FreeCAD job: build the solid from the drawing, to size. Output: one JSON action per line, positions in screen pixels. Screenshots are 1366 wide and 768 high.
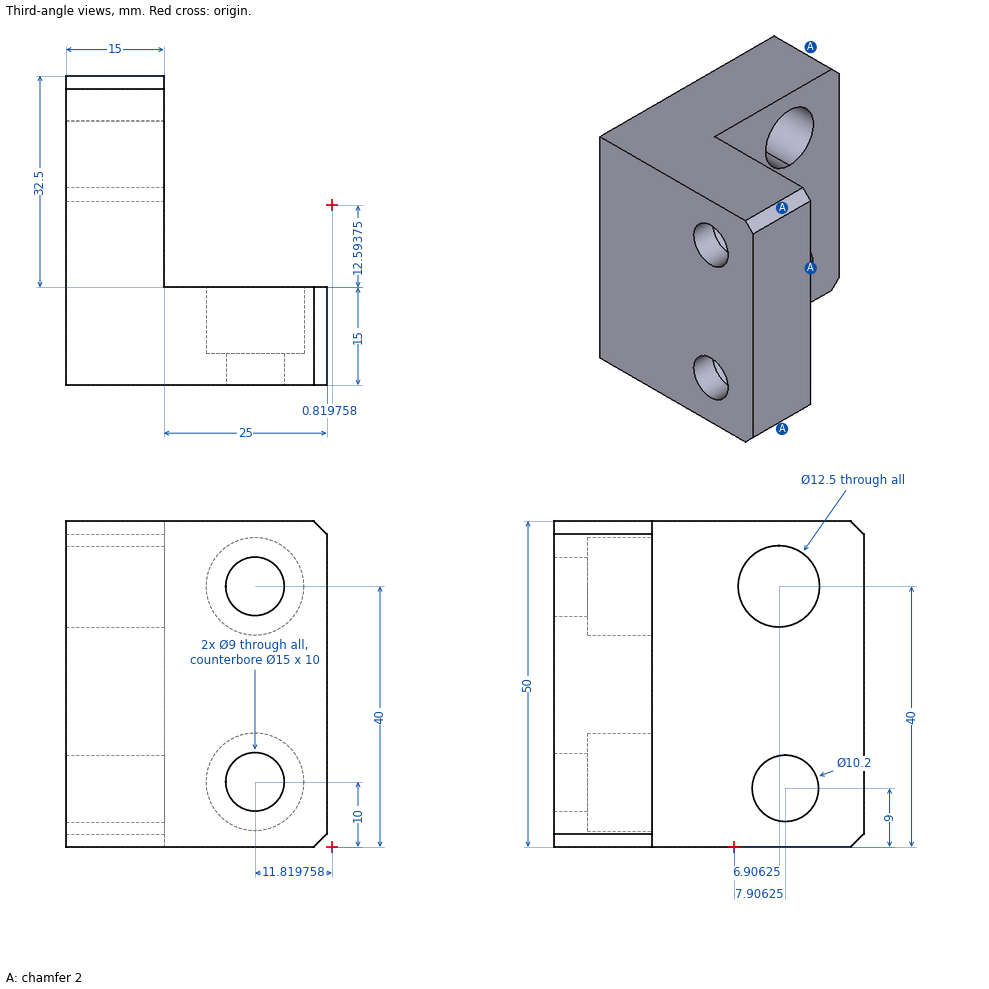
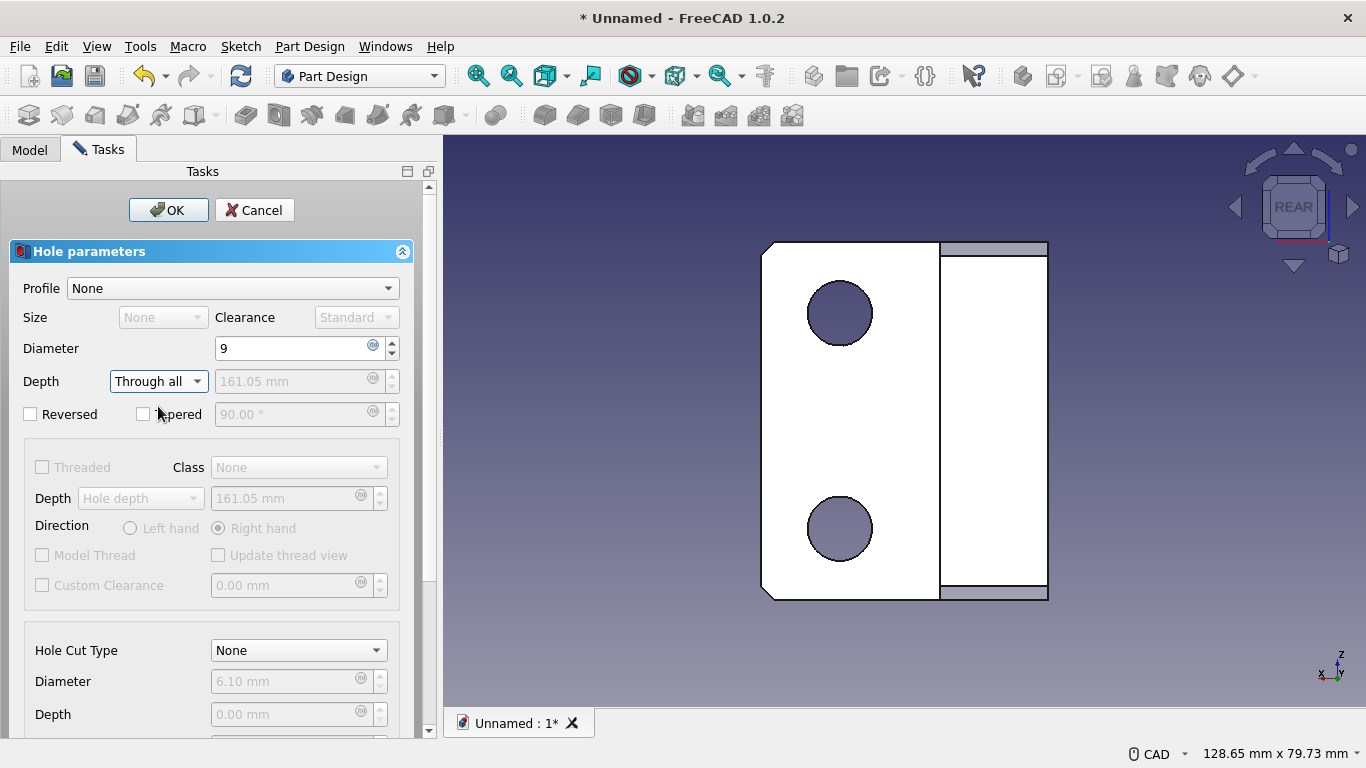
{"action": "left_click", "coordinate": [300, 650]}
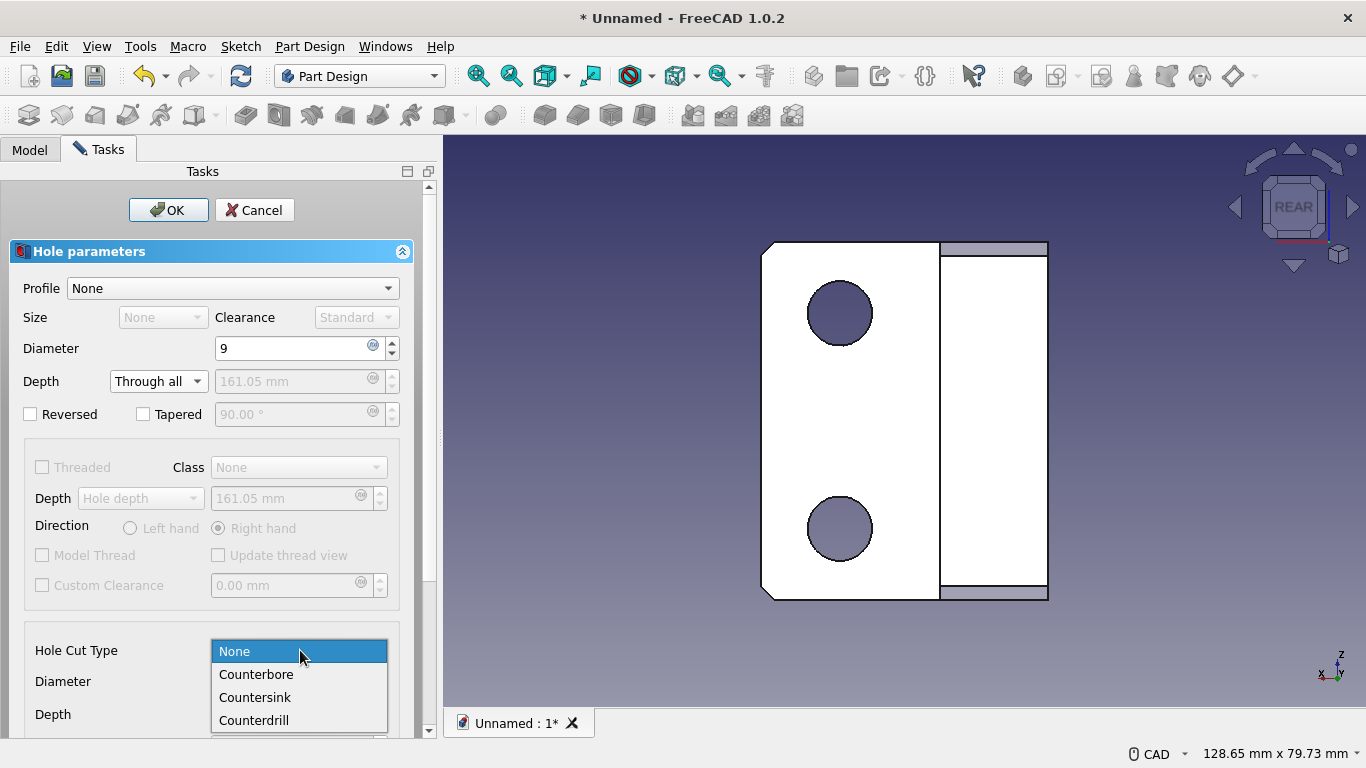
{"action": "left_click", "coordinate": [298, 674]}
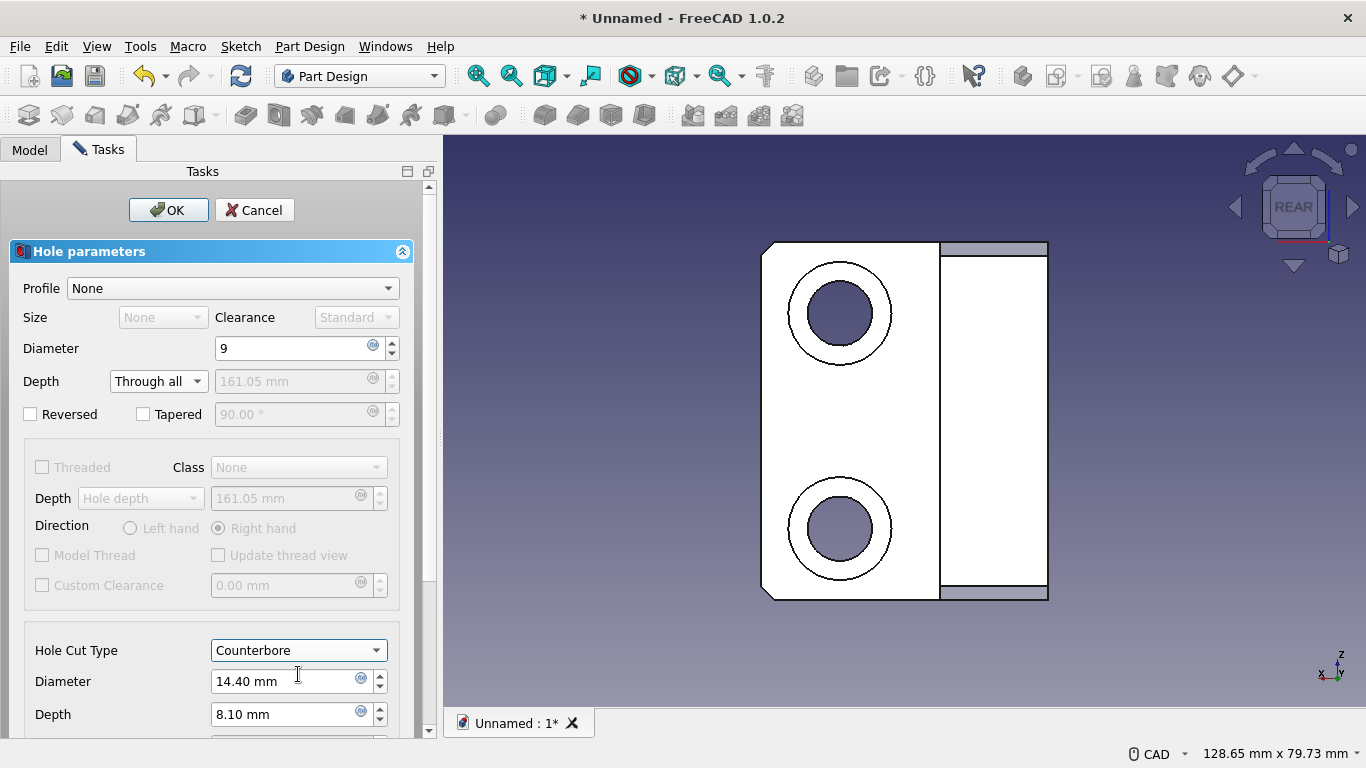
{"action": "triple_click", "coordinate": [292, 682]}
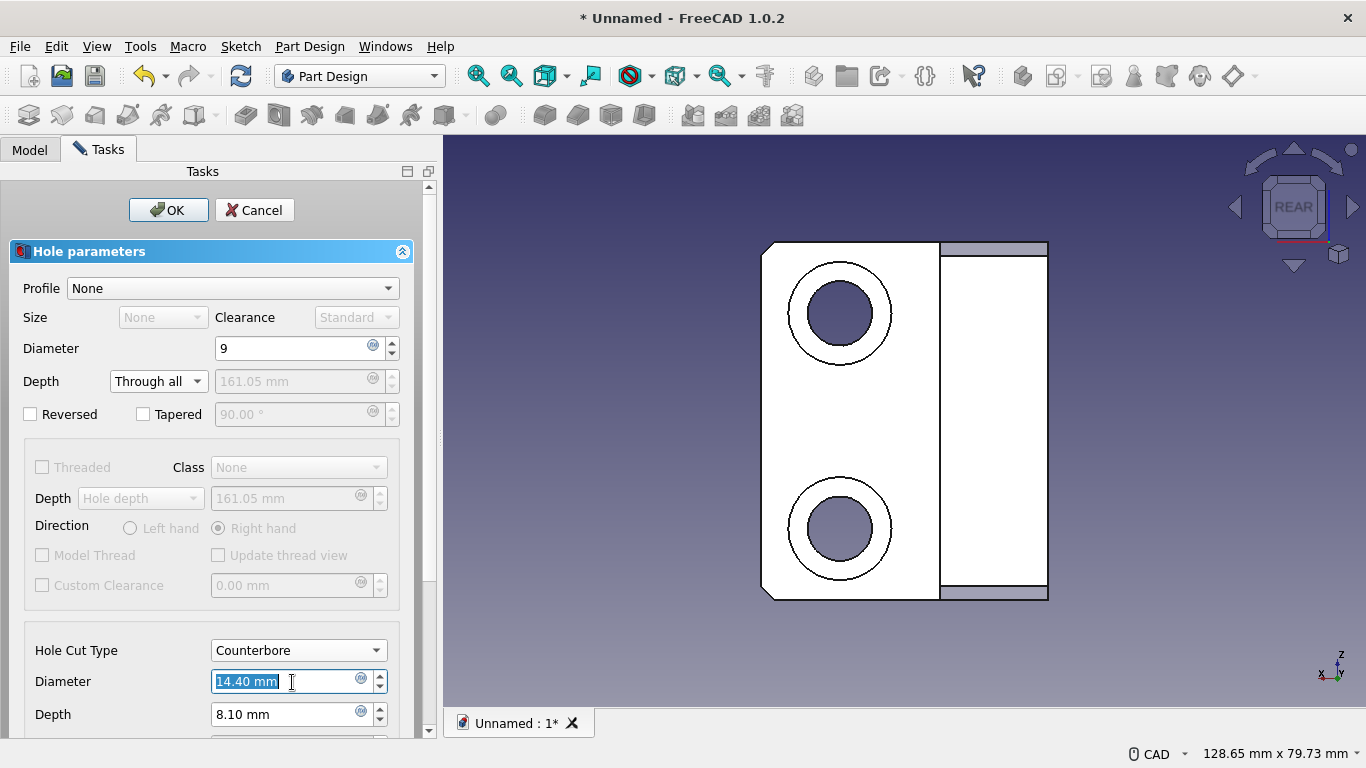
{"action": "type", "text": "15"}
{"action": "key", "text": "Tab"}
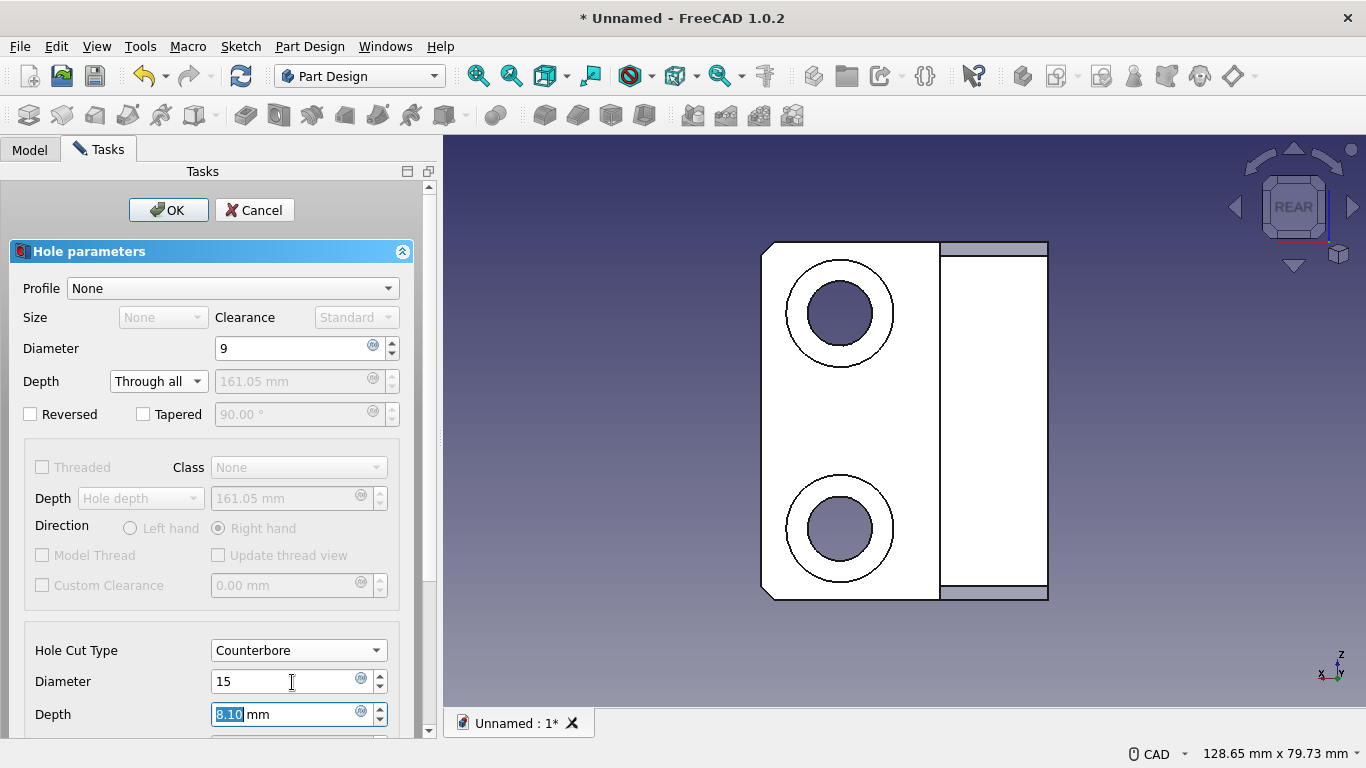
{"action": "type", "text": "10"}
{"action": "key", "text": "Tab"}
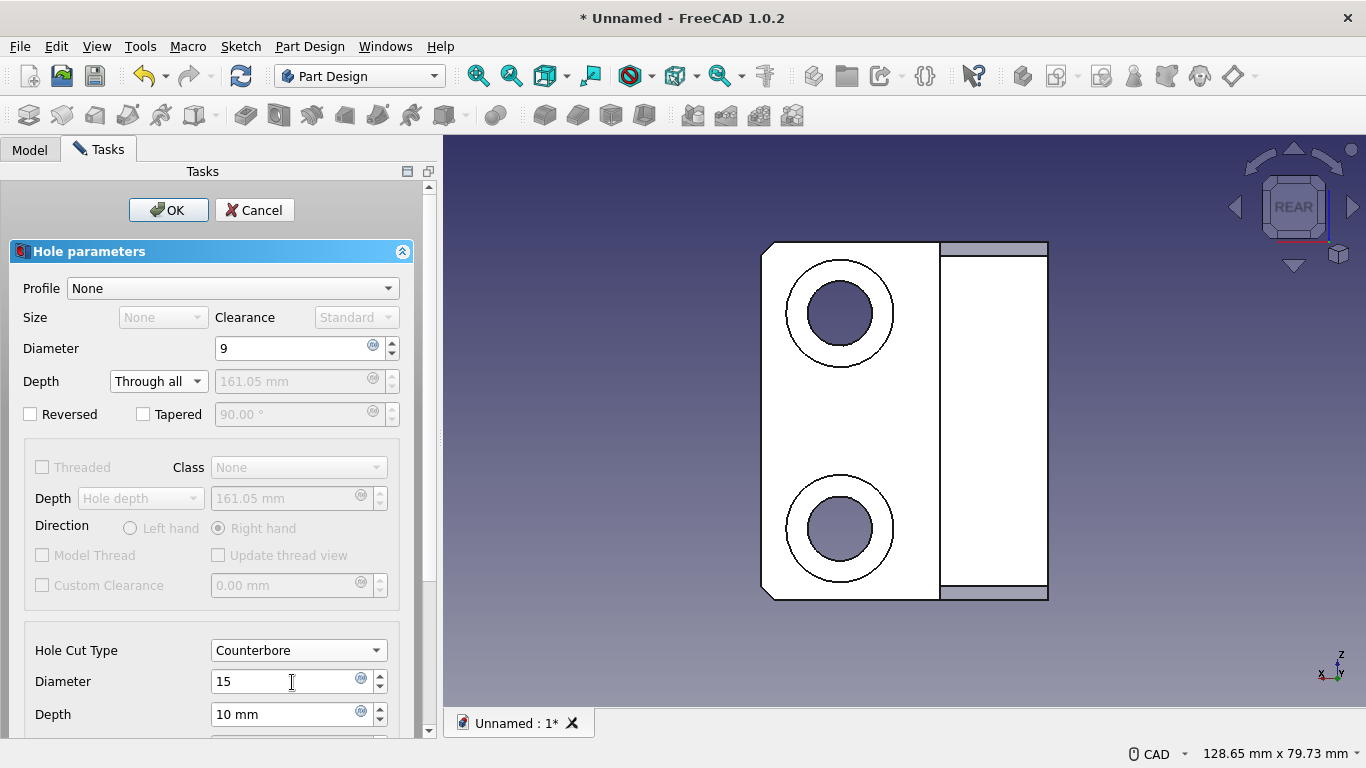
{"action": "left_click", "coordinate": [169, 210]}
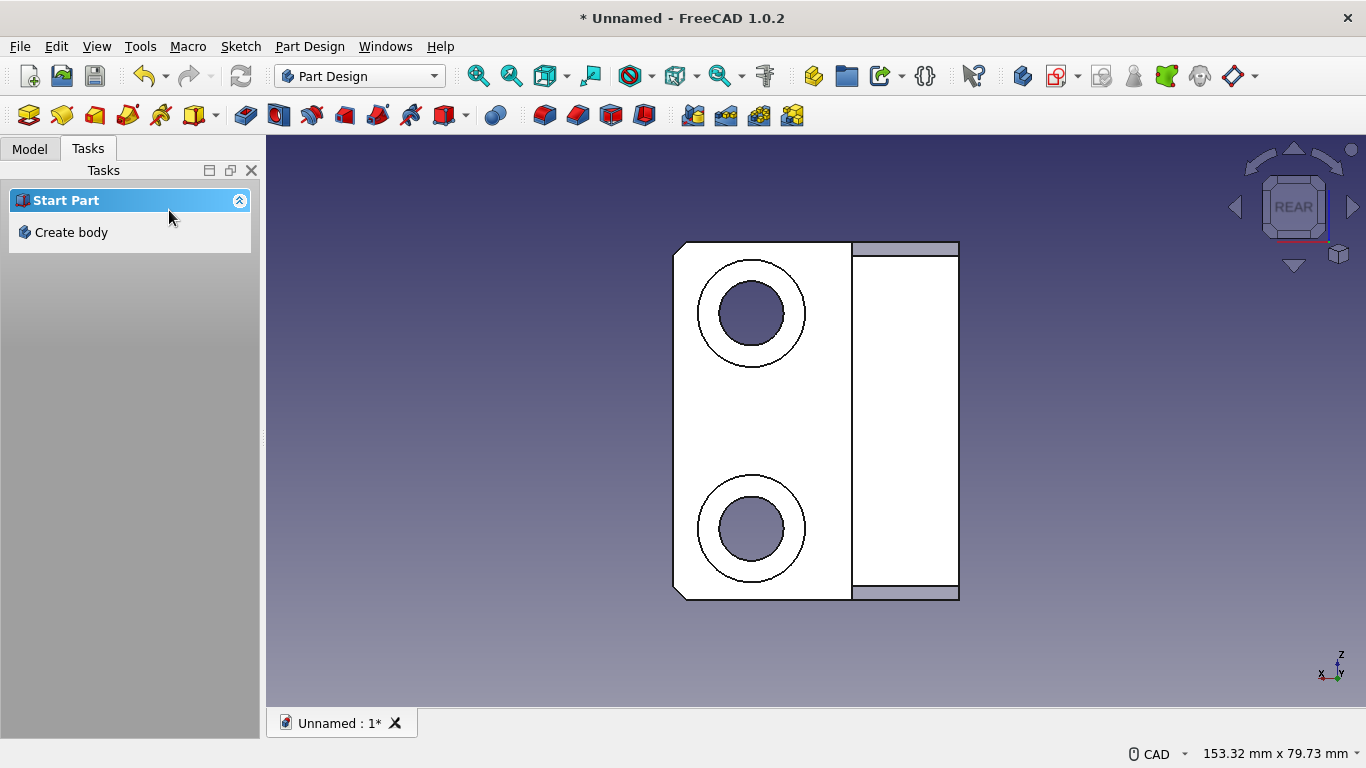
{"action": "key", "text": "0"}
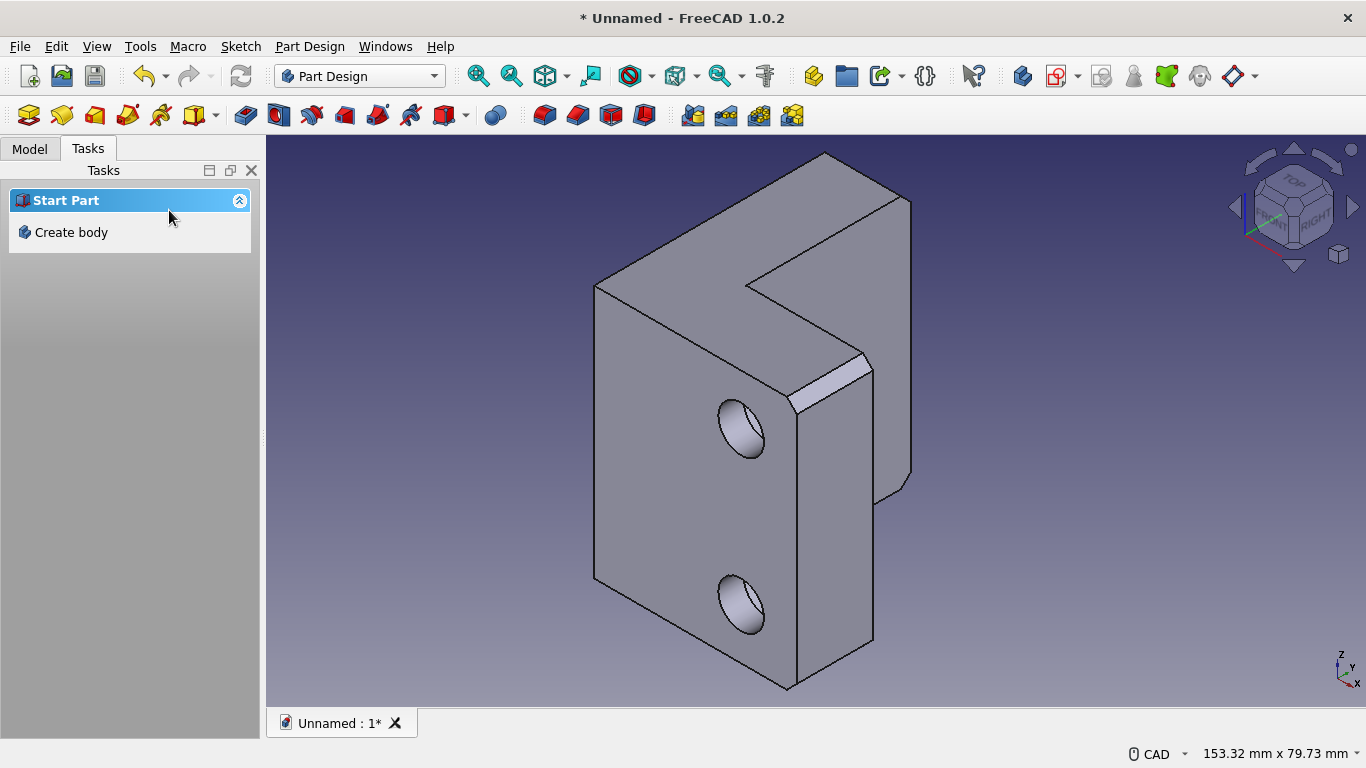
{"action": "left_click", "coordinate": [852, 328]}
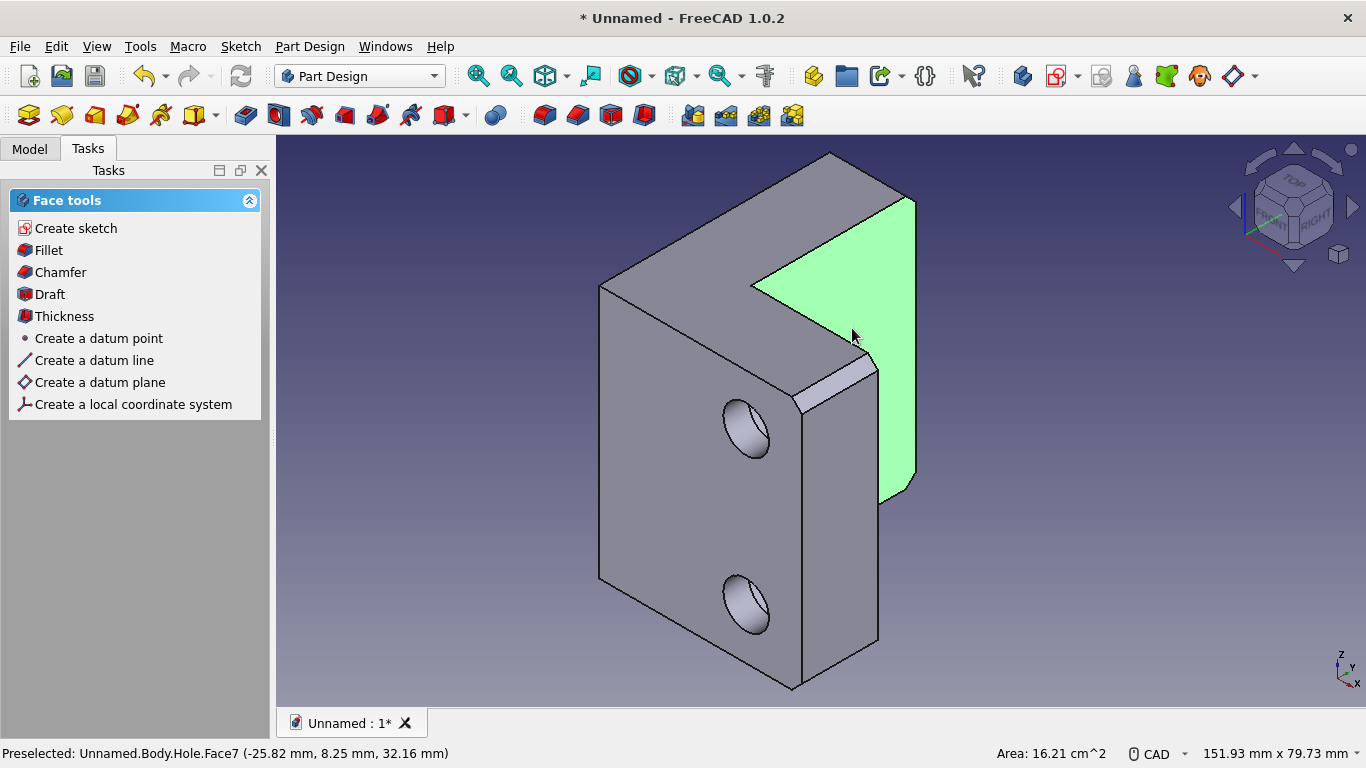
{"action": "left_click", "coordinate": [1056, 76]}